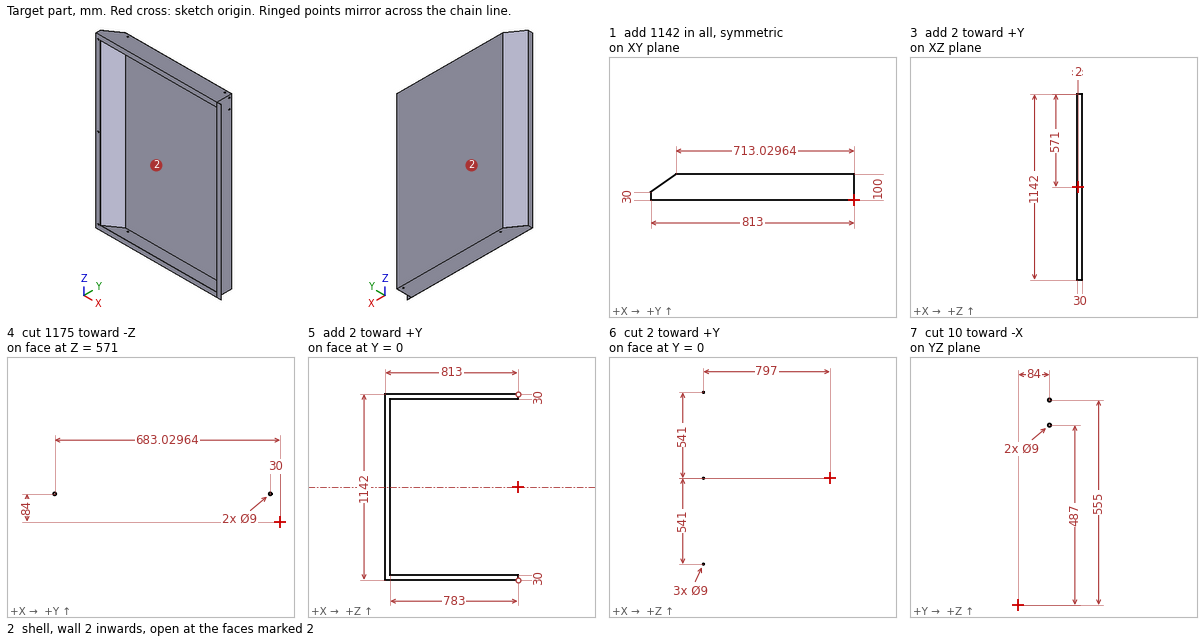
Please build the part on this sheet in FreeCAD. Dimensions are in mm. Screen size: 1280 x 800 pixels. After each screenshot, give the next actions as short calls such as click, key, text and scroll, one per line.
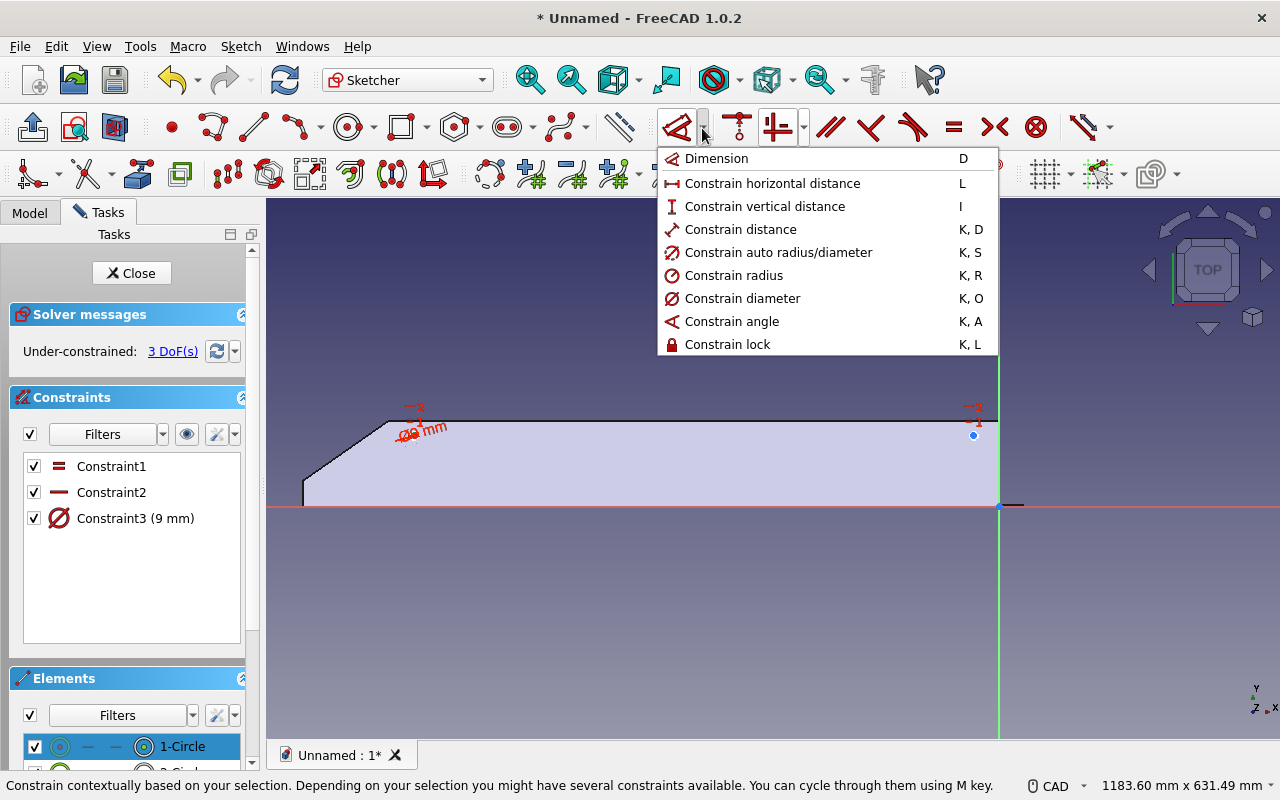
click(828, 206)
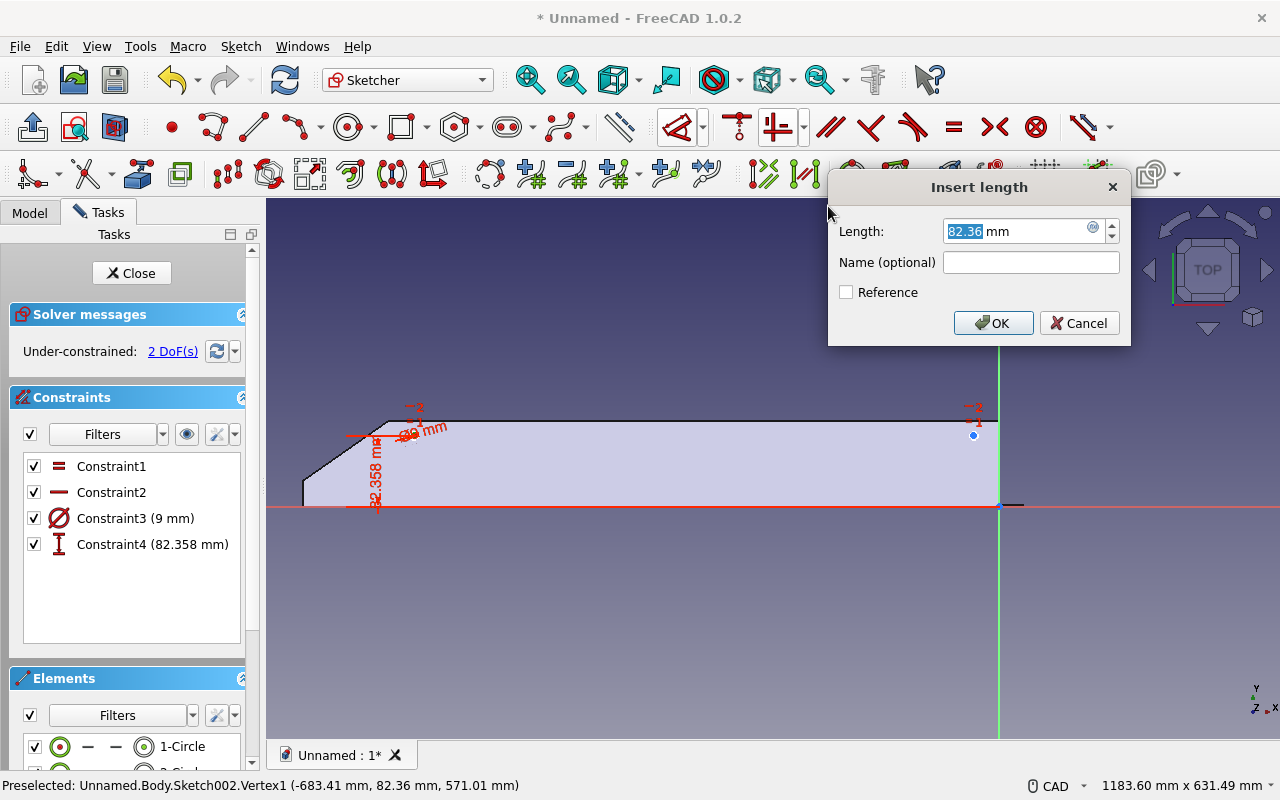
text(84)
key(Return)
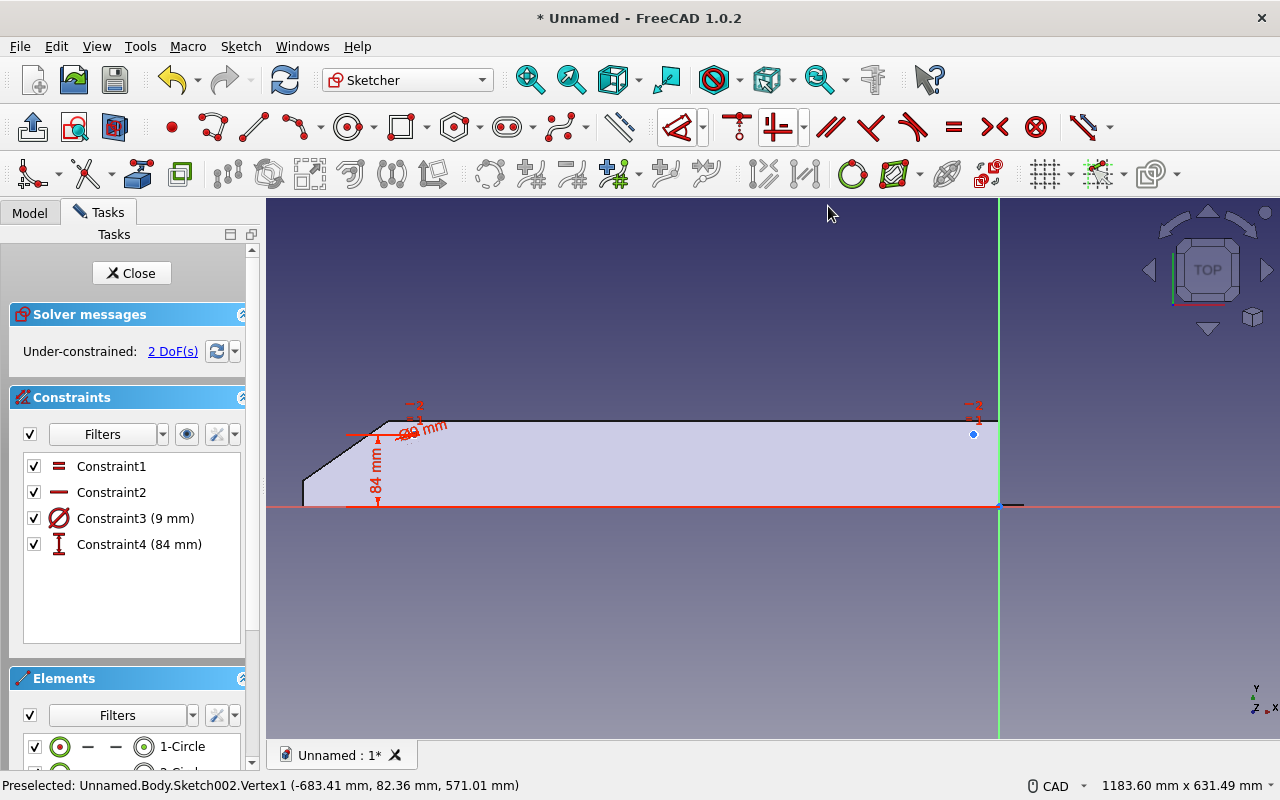
scroll(974, 435, up, 3)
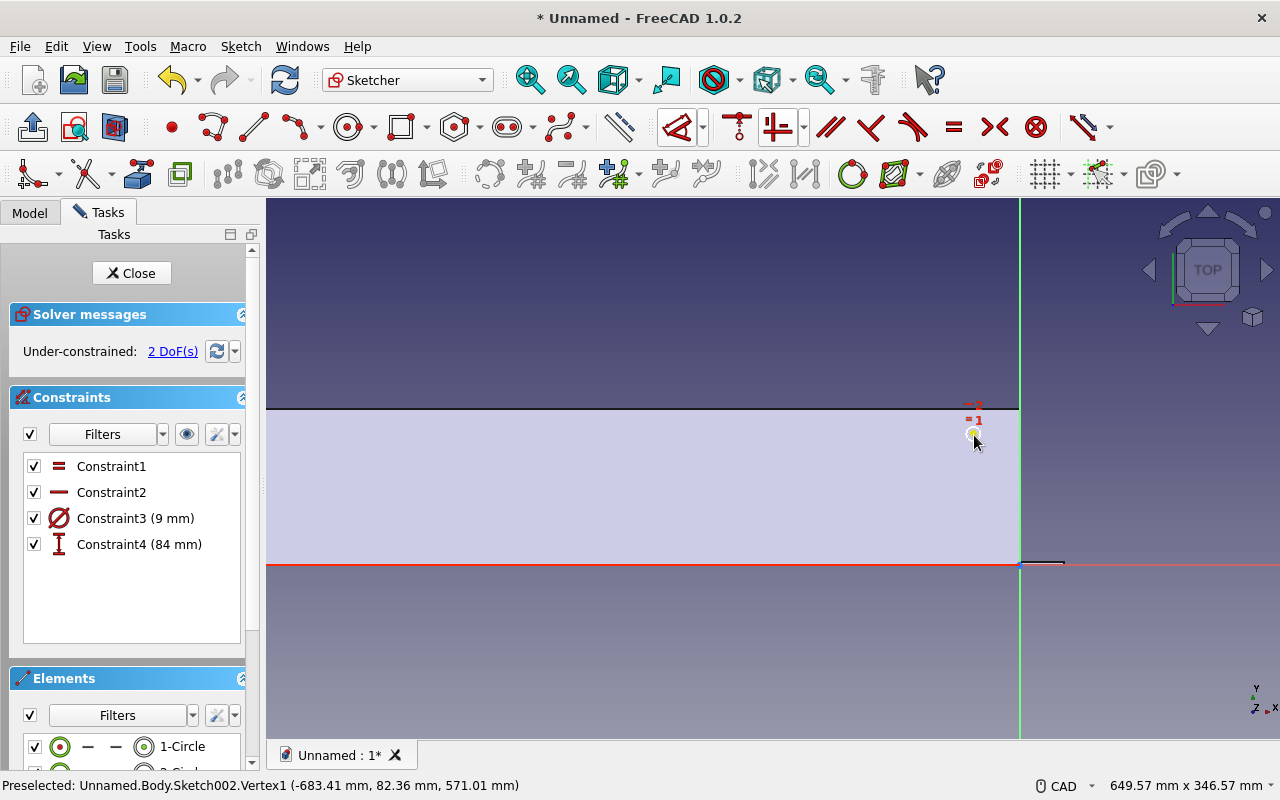
click(973, 434)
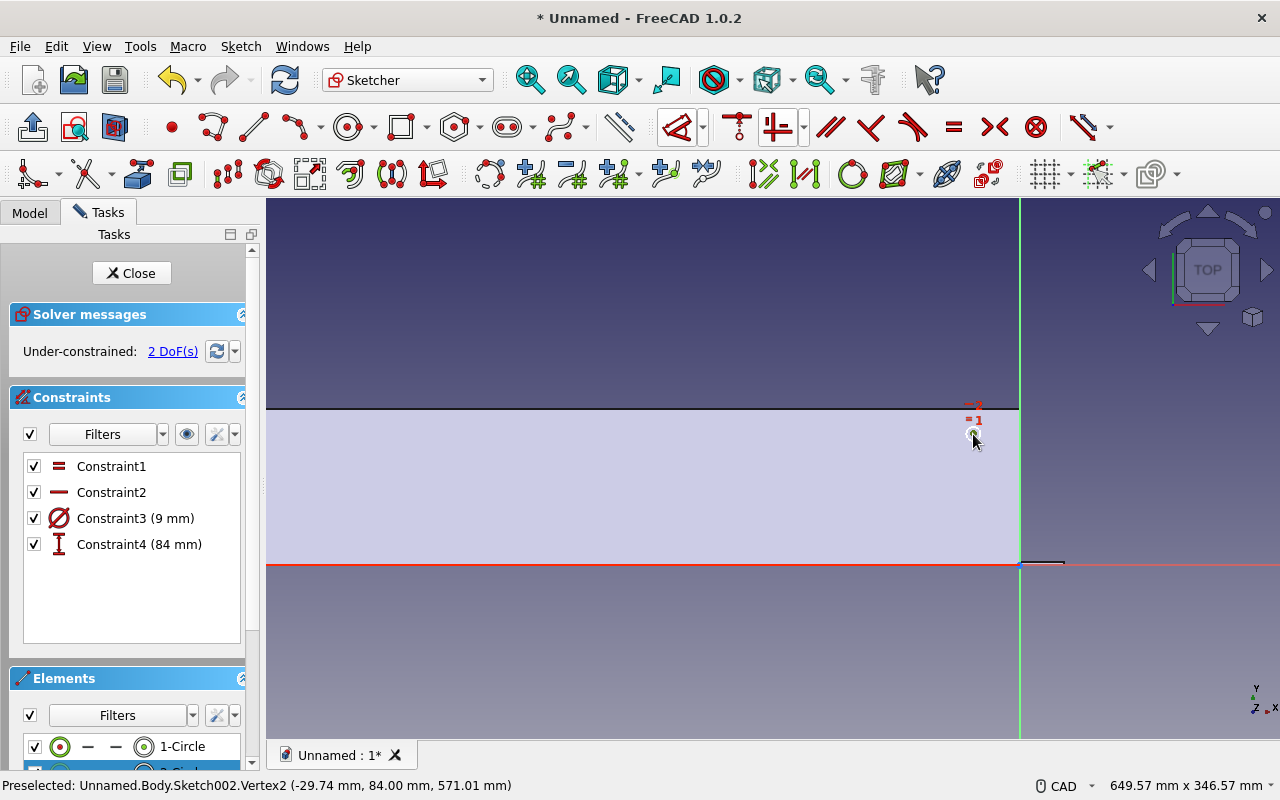
key(l)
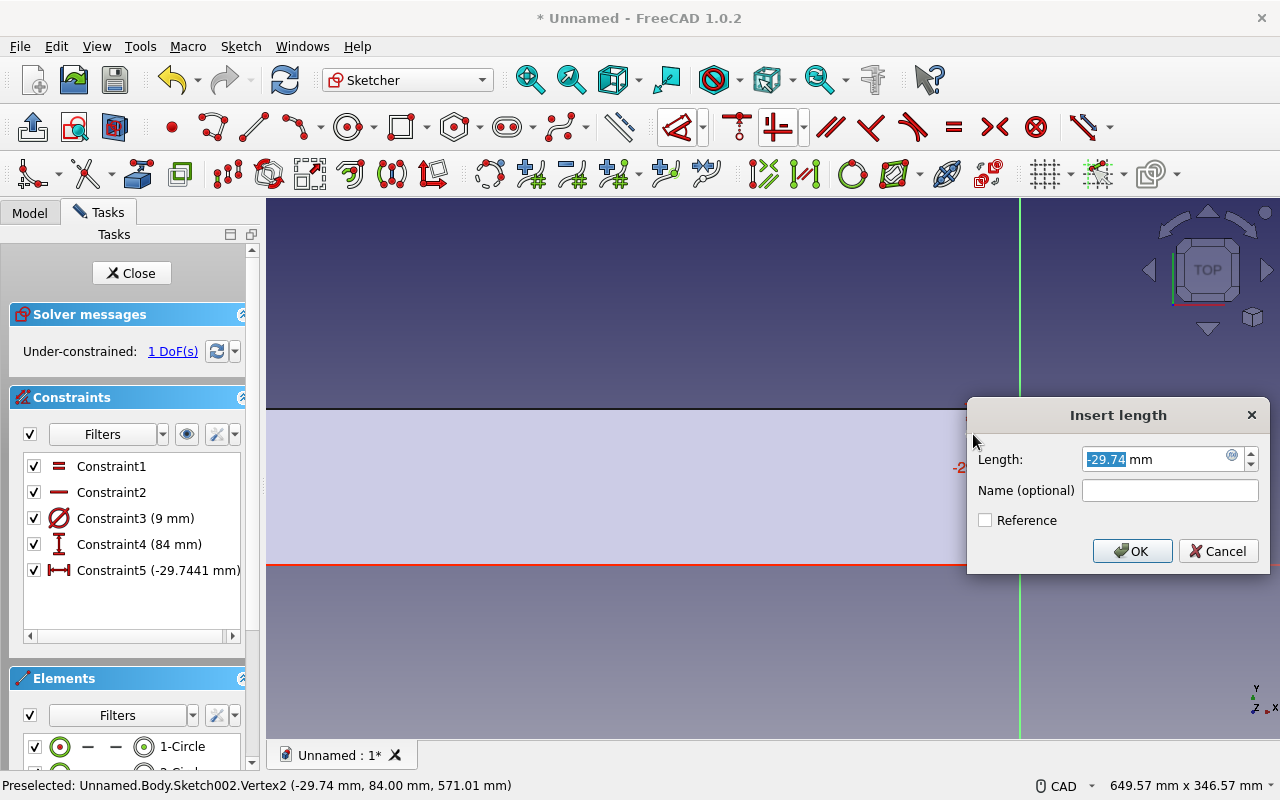
text(-30)
key(Return)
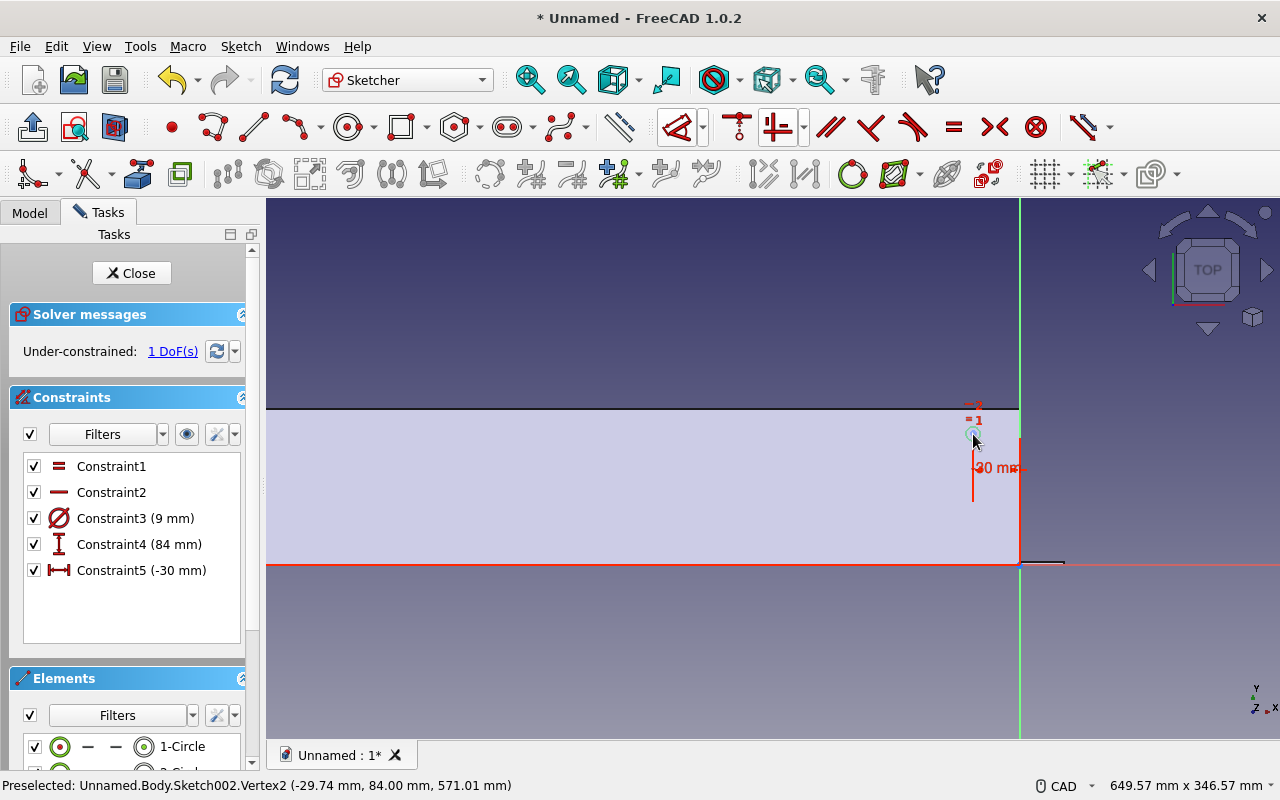
scroll(974, 435, down, 3)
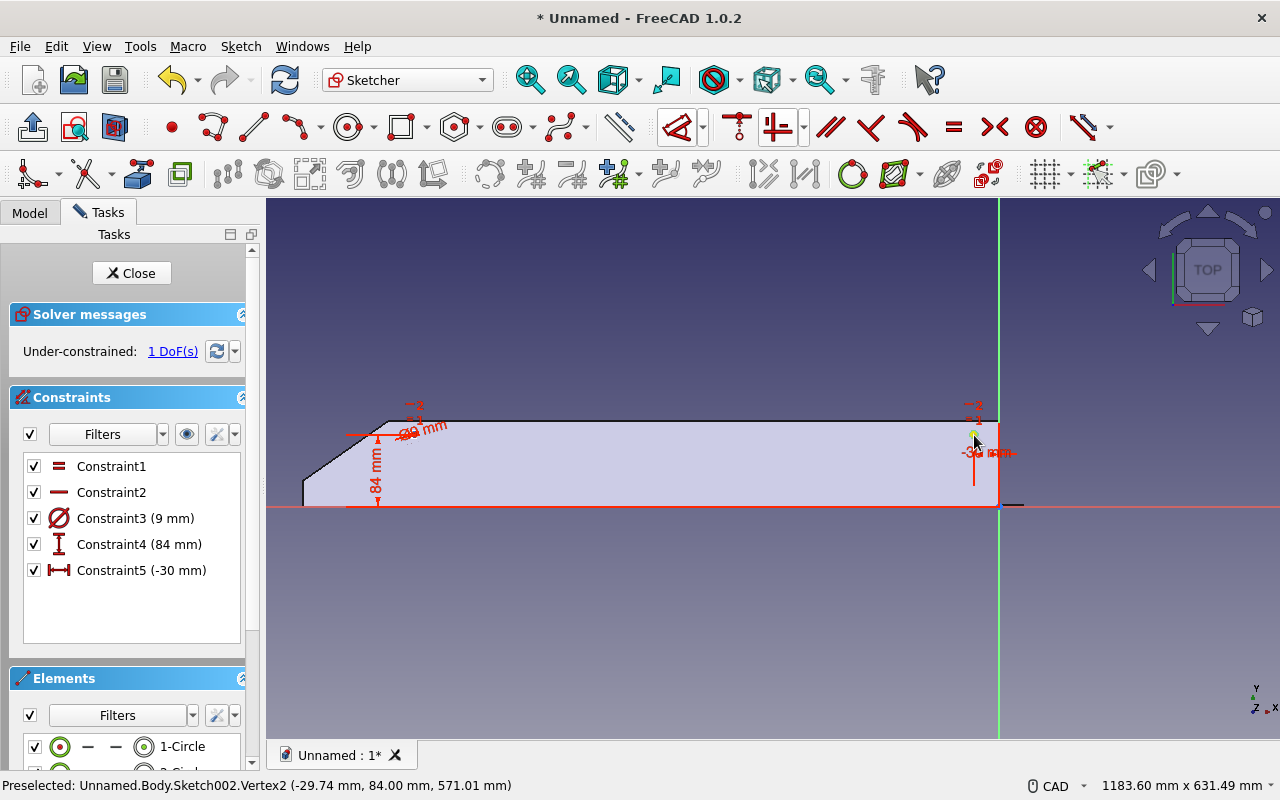
click(414, 435)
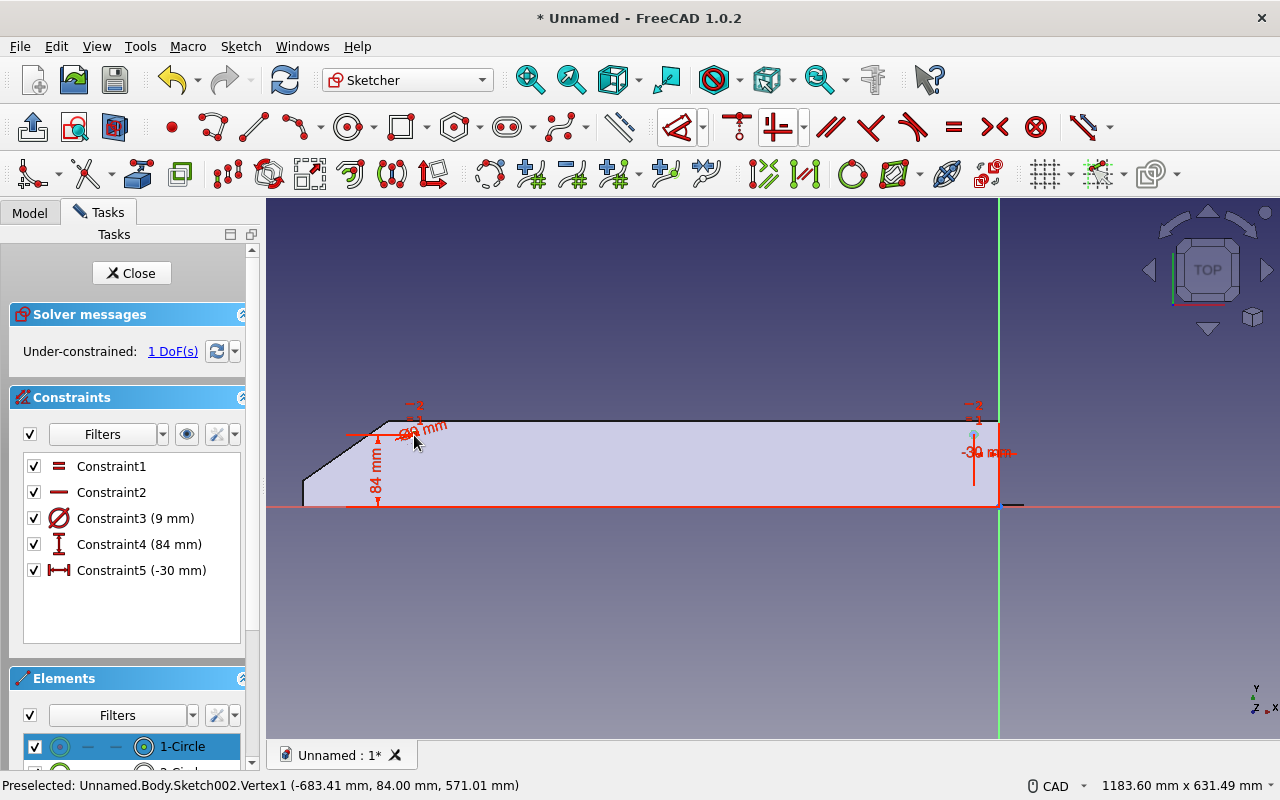
key(l)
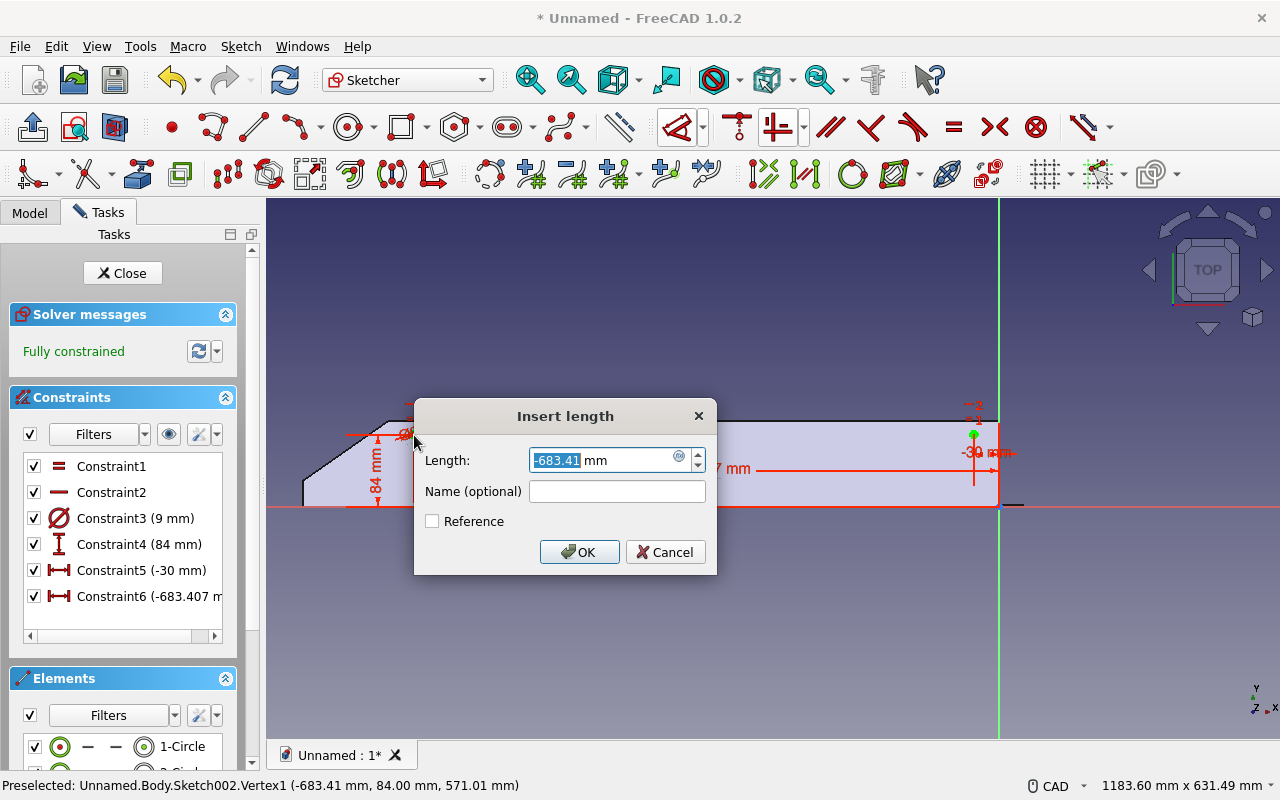
text(-683.02964)
key(Return)